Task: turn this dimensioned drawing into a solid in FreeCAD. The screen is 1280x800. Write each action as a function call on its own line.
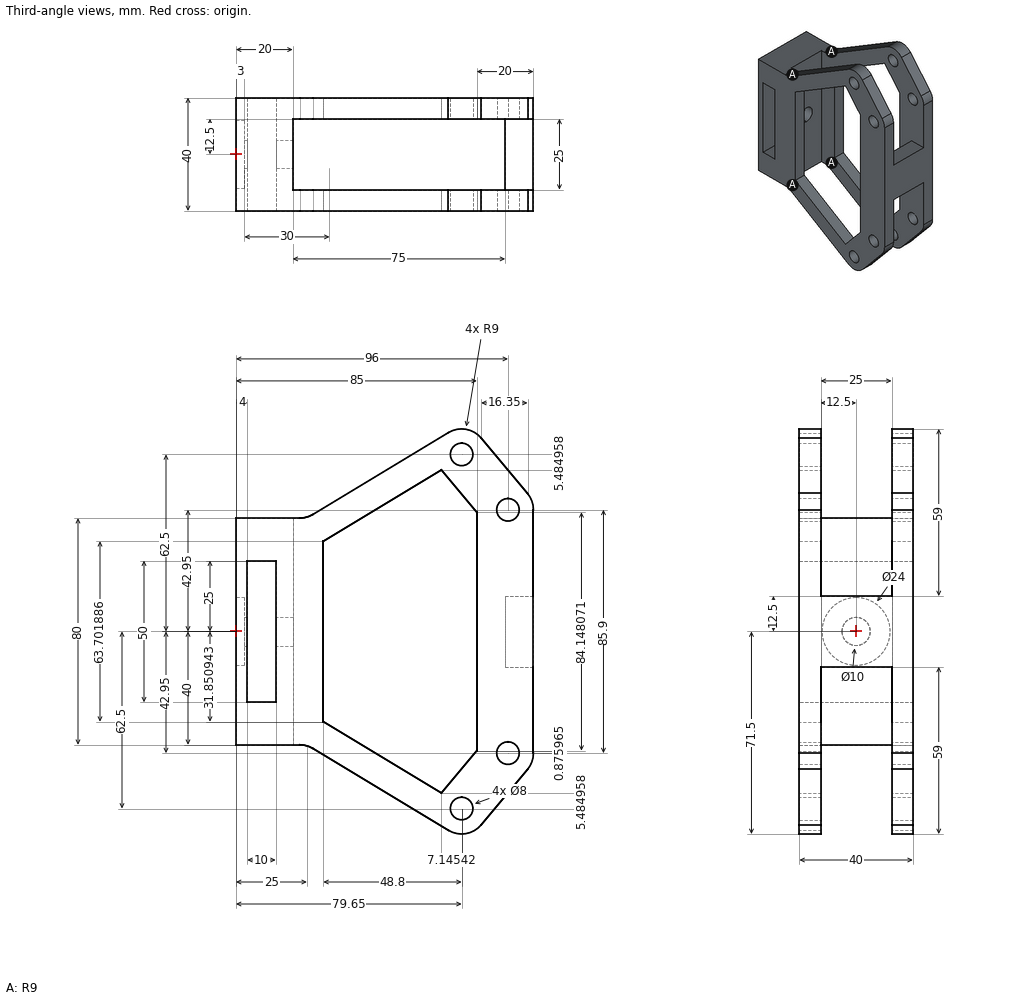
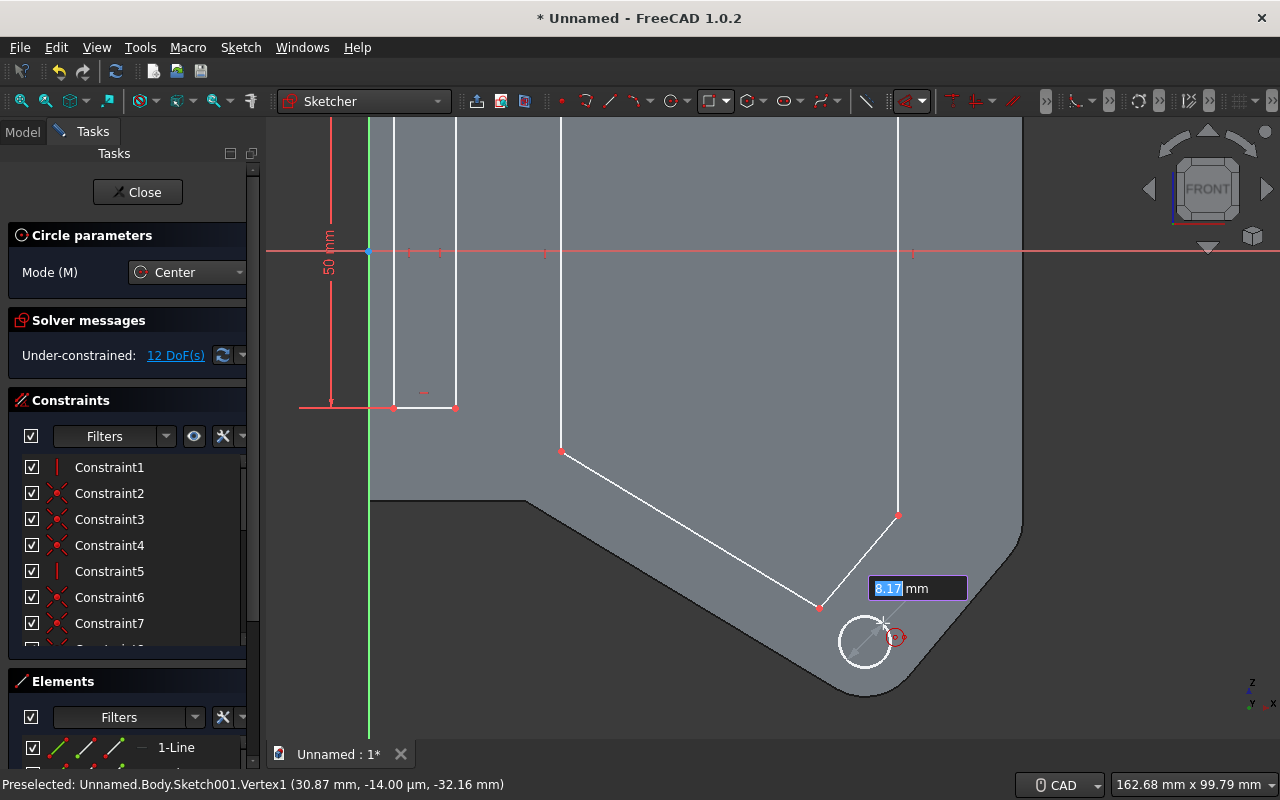
text(8)
key(Return)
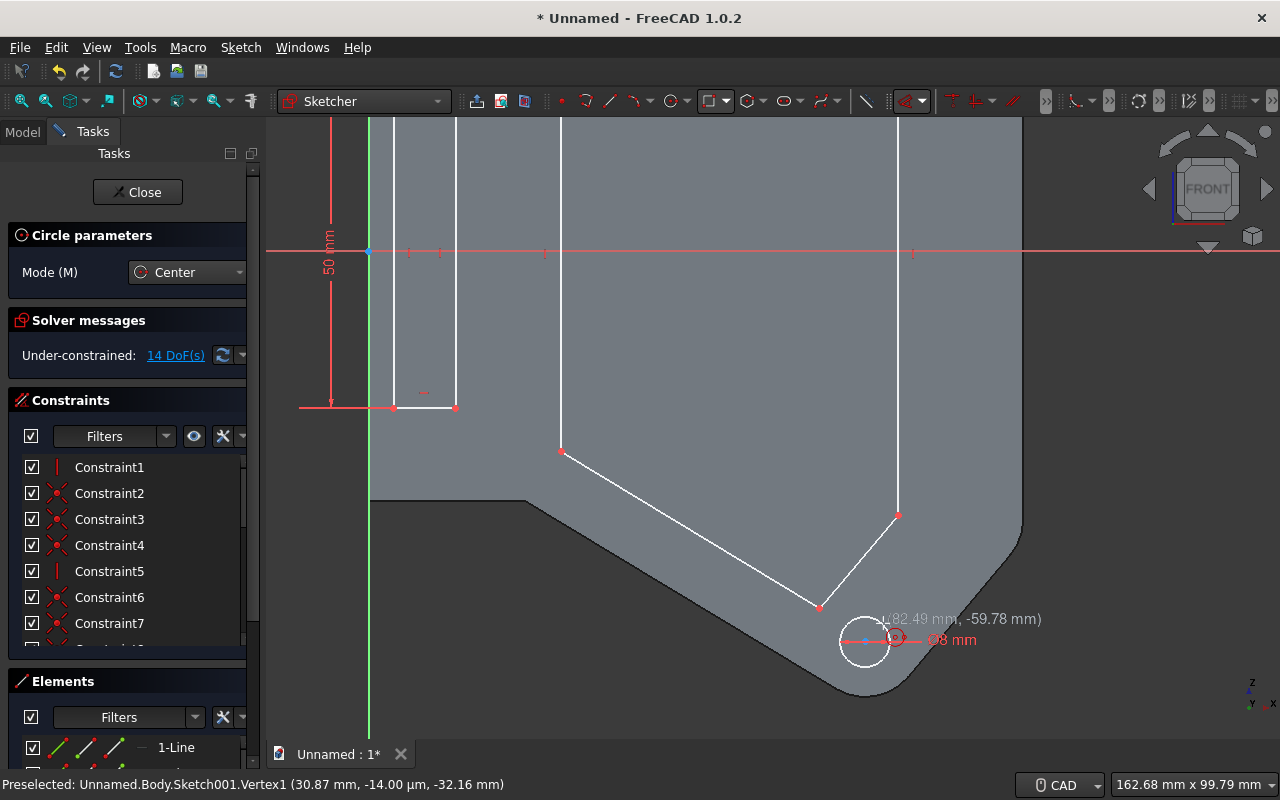
click(967, 519)
move(985, 501)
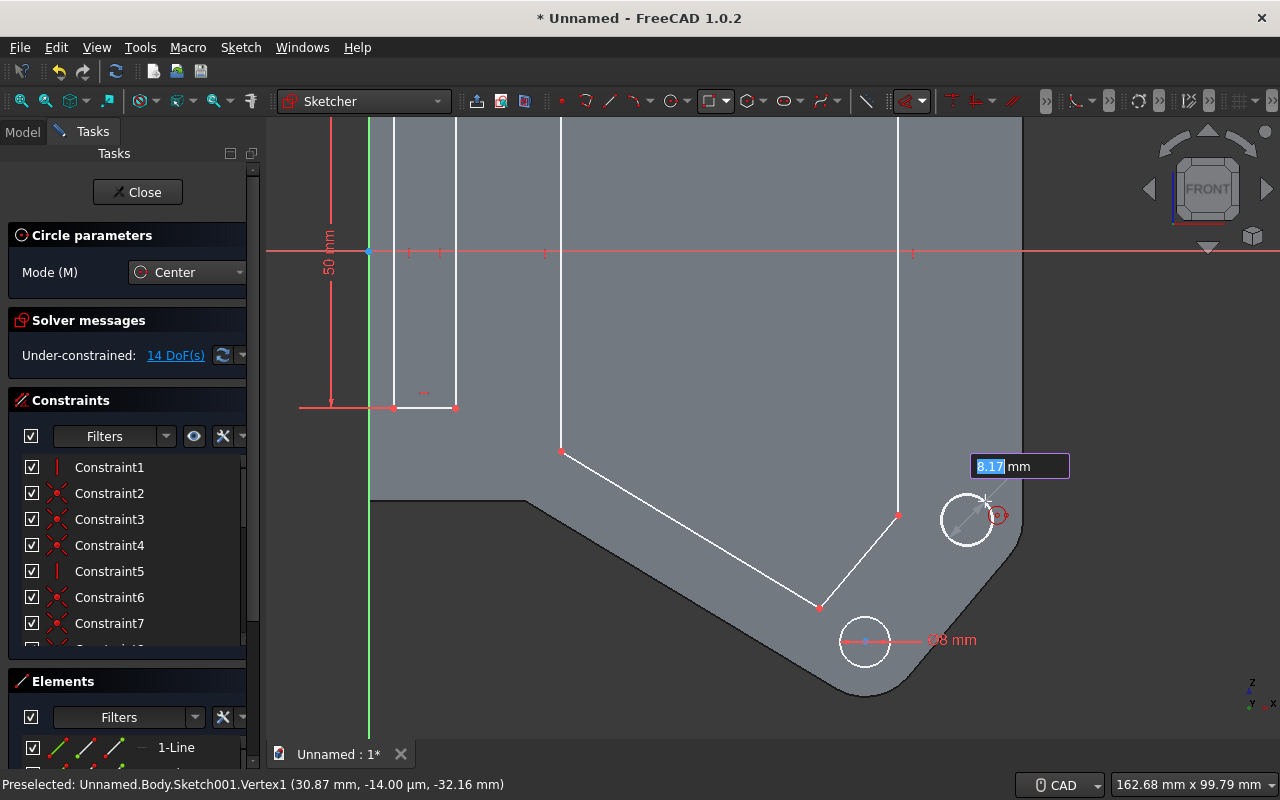
text(8)
key(Return)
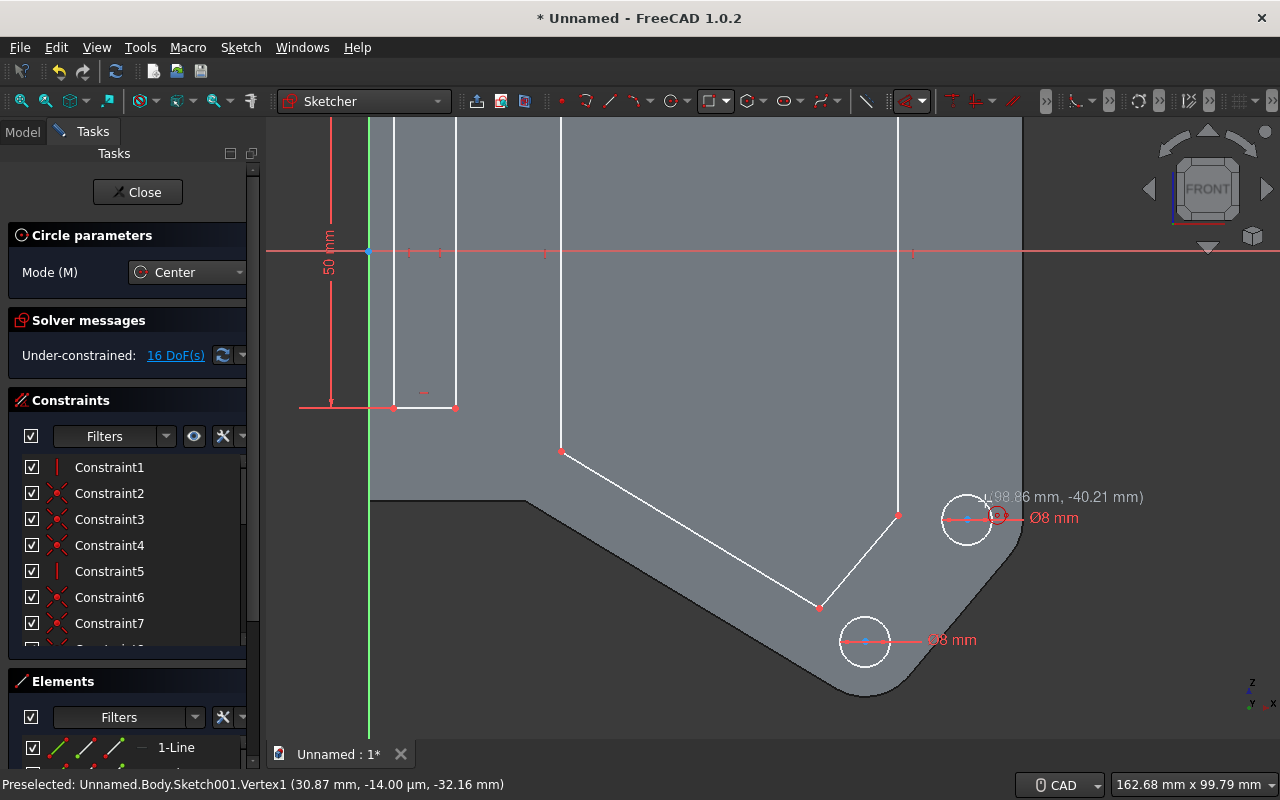
scroll(724, 572, down, 4)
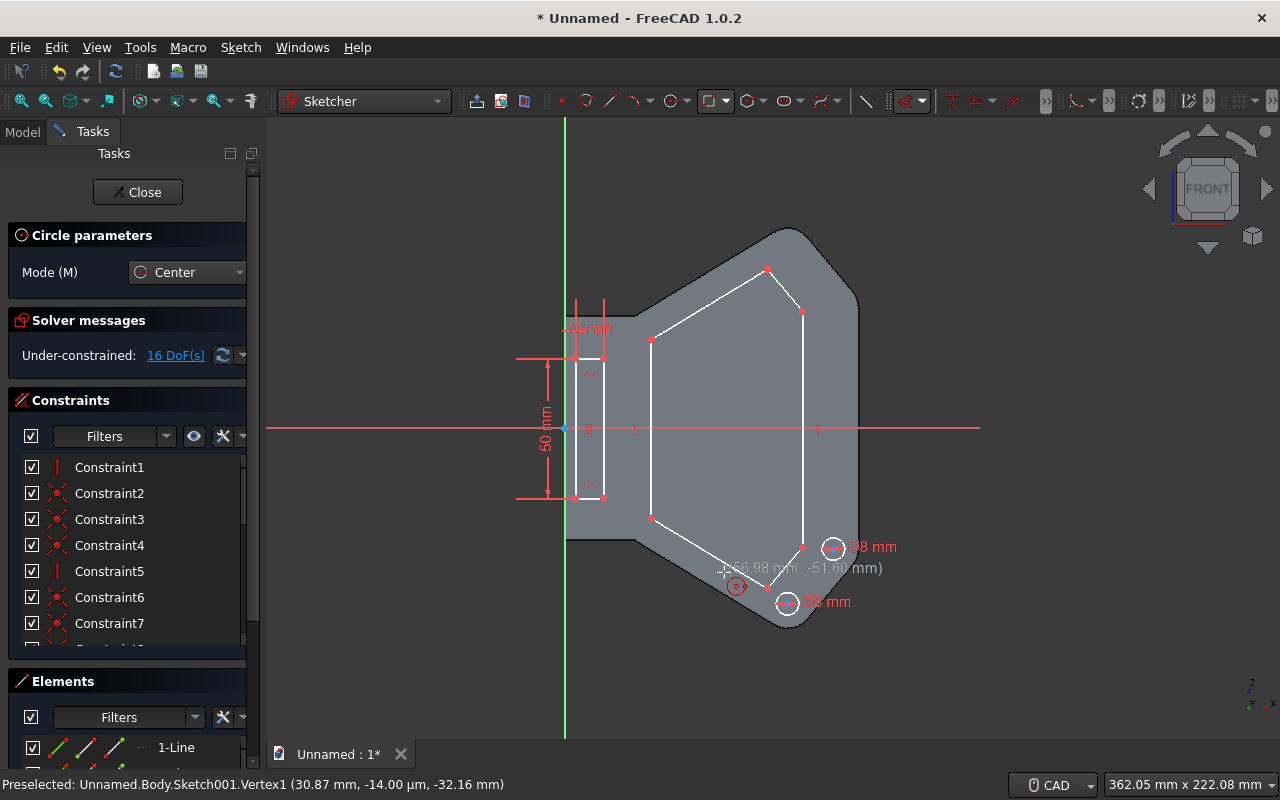
scroll(834, 308, up, 4)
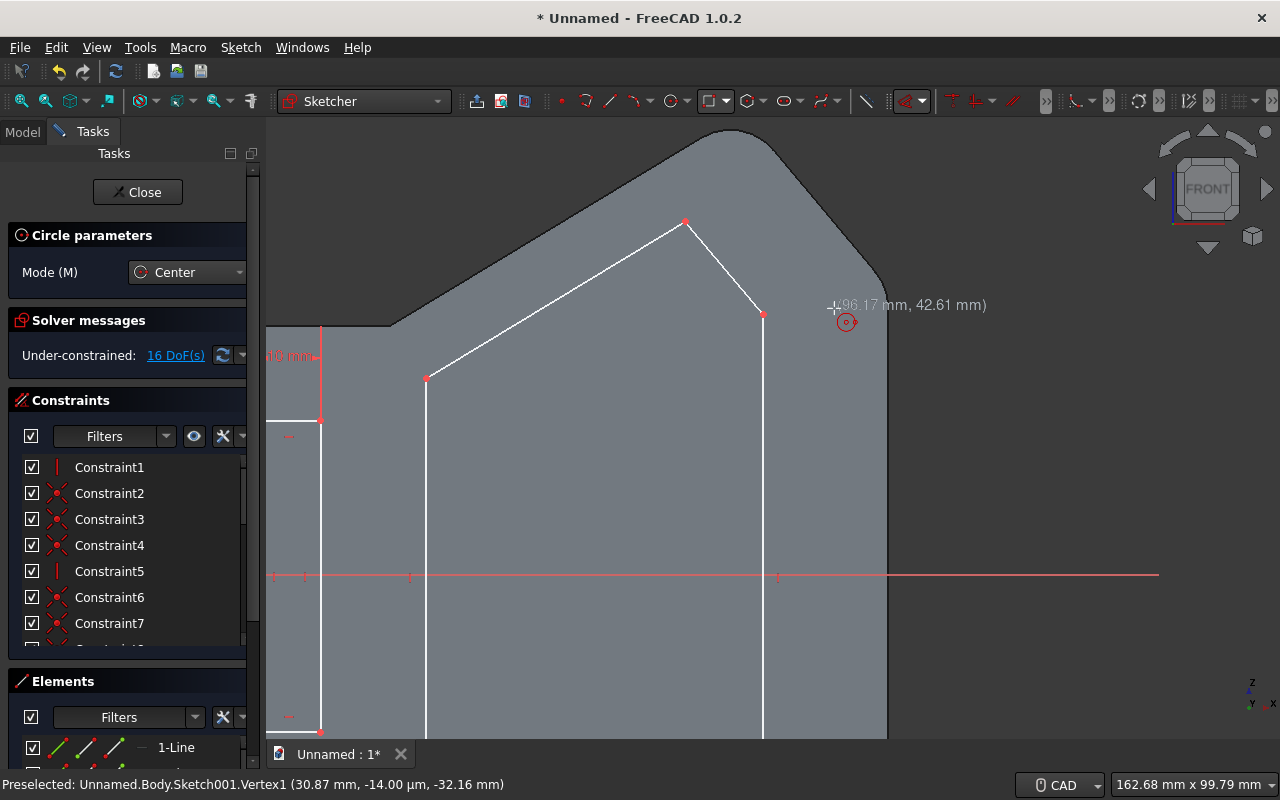
click(832, 308)
move(850, 290)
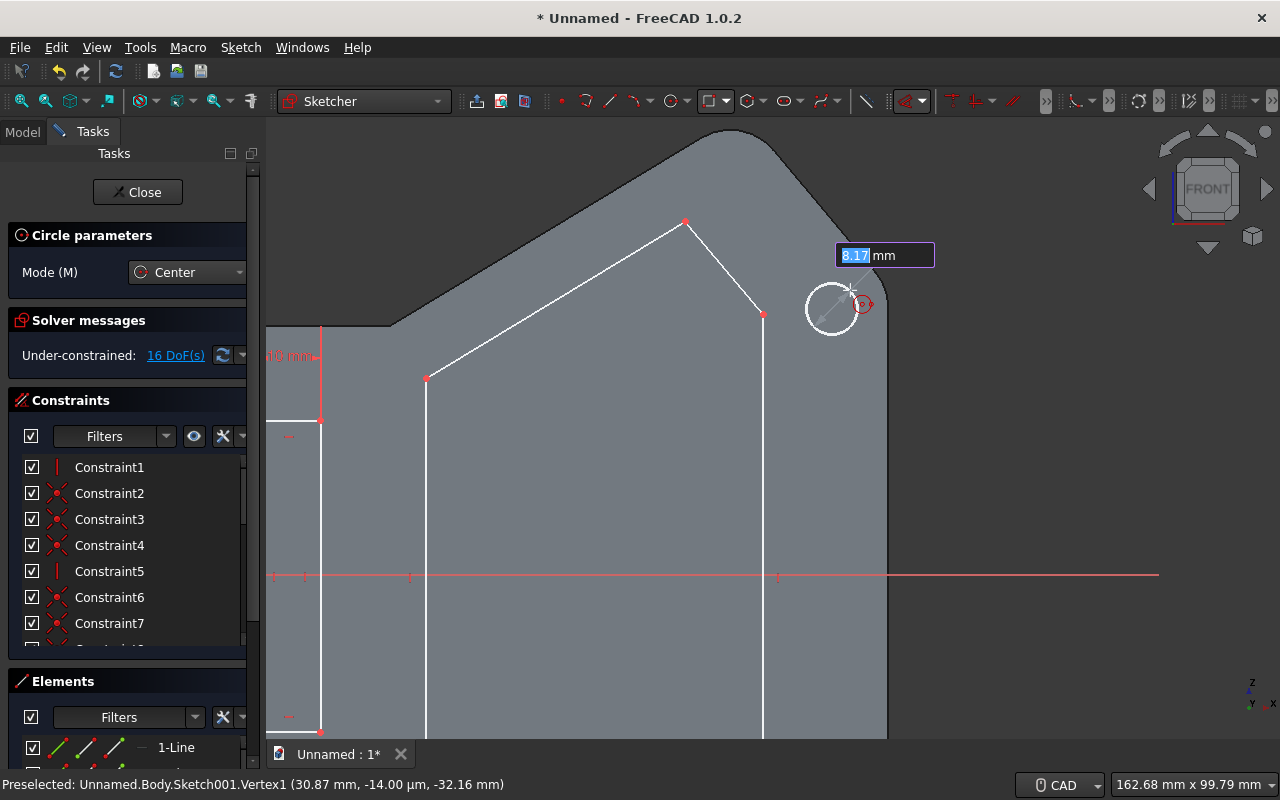
text(8)
key(Return)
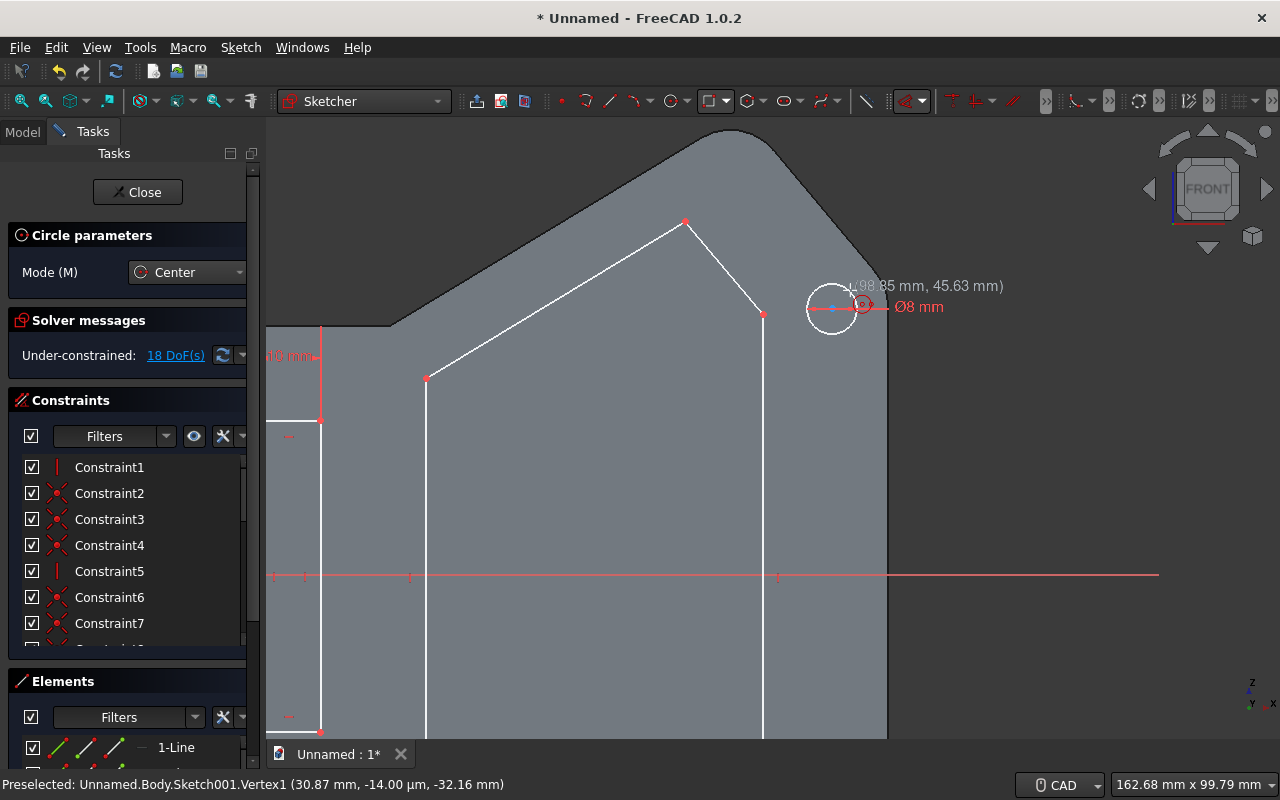
click(730, 186)
move(748, 168)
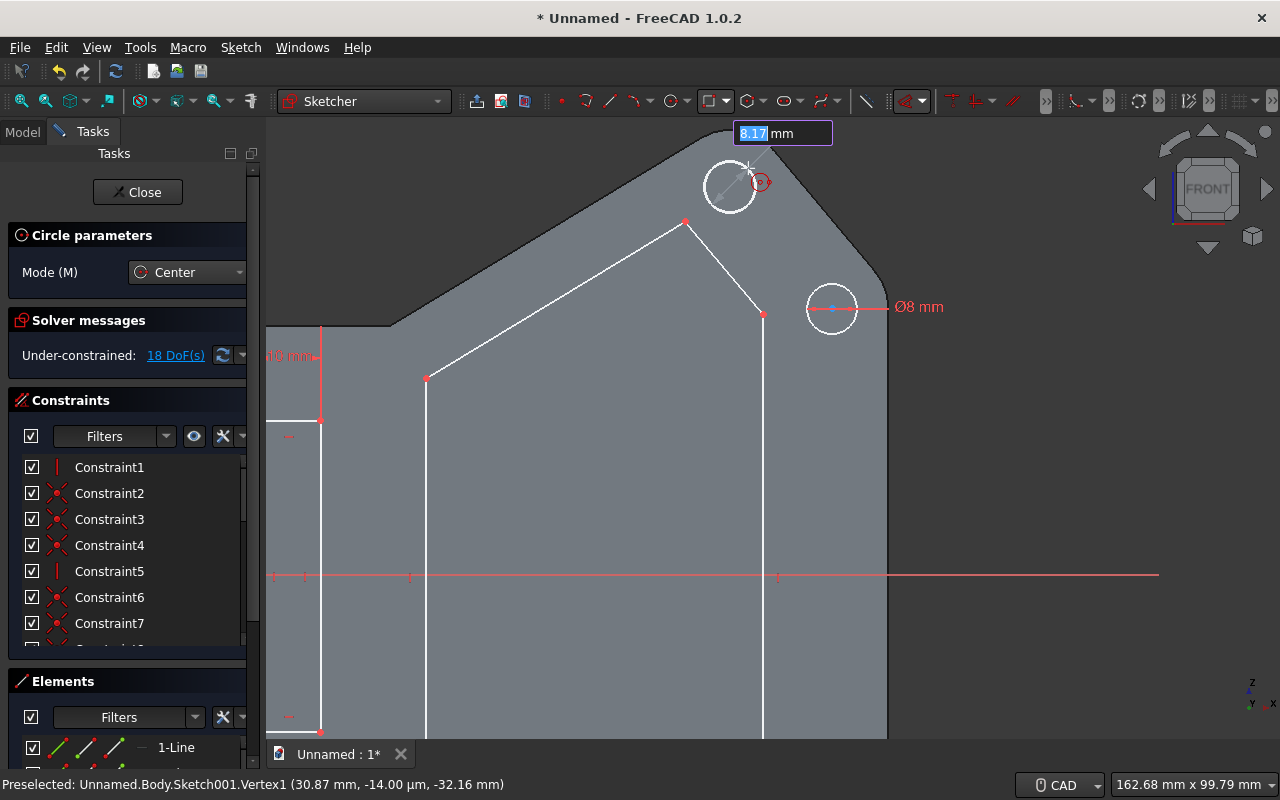
text(8)
key(Return)
key(Escape)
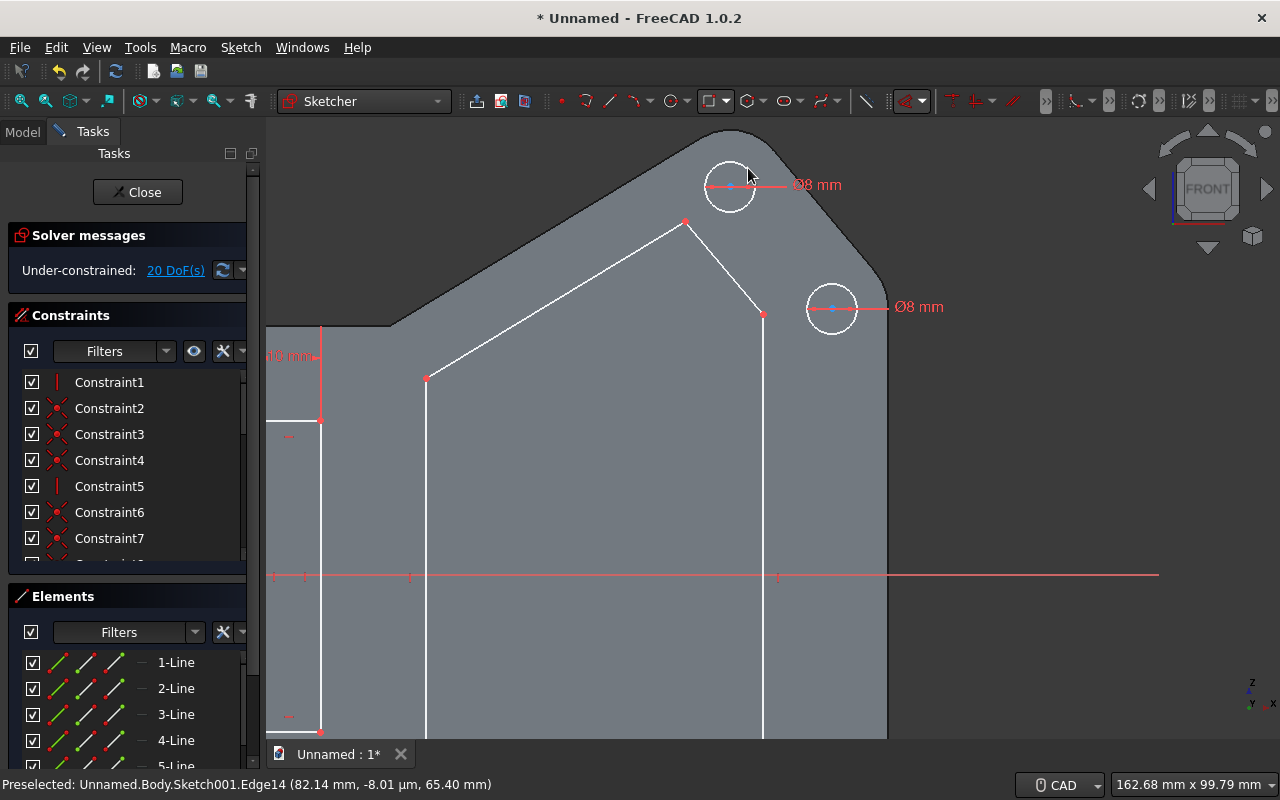
scroll(834, 308, down, 4)